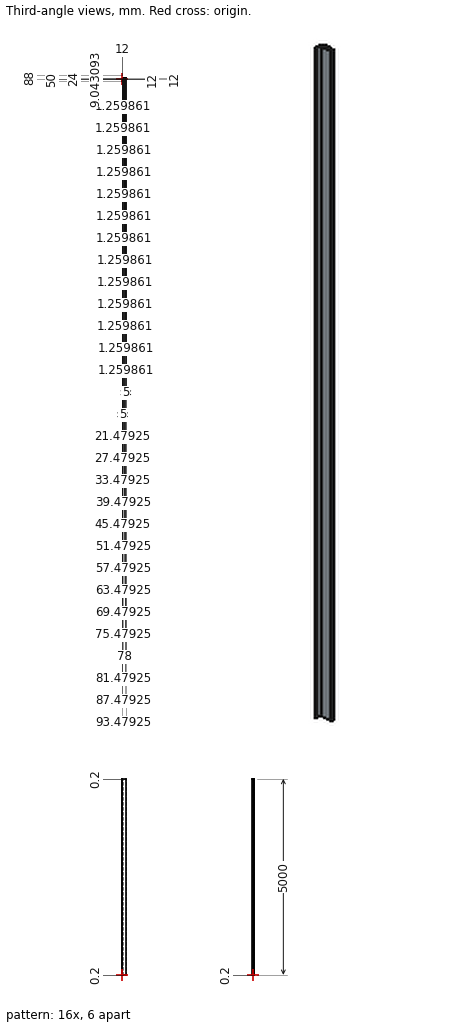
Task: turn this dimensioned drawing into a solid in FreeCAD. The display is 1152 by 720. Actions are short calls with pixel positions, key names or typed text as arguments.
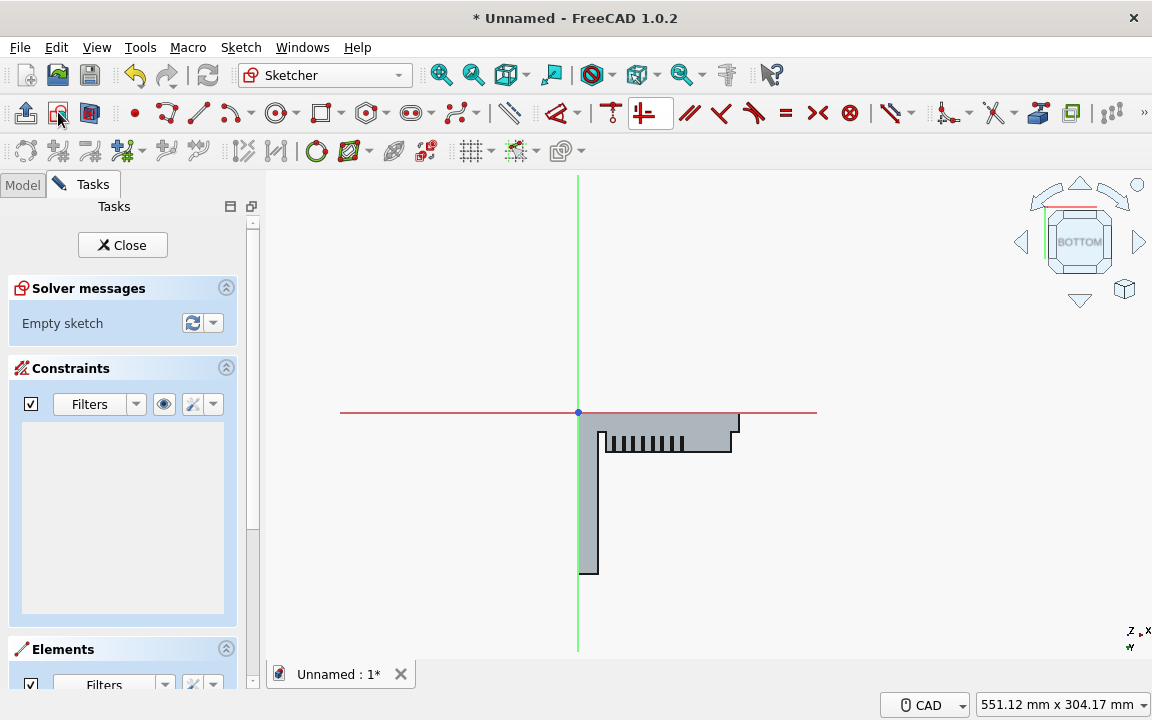
scroll(694, 446, up, 15)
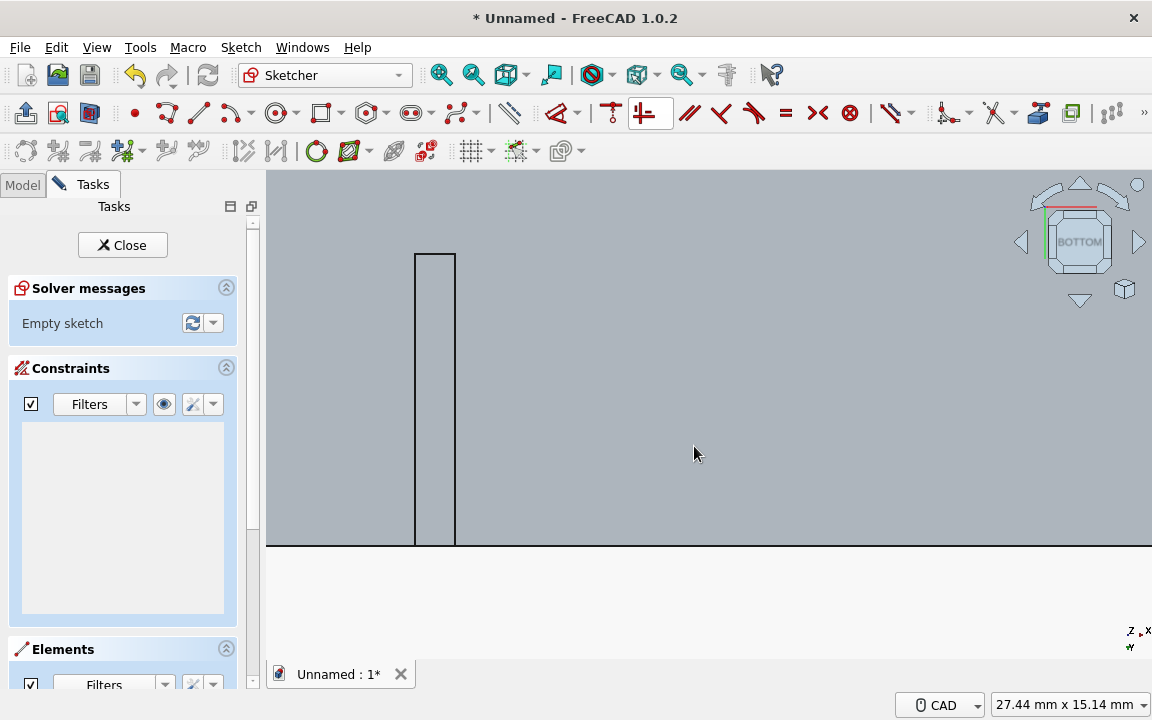
click(322, 114)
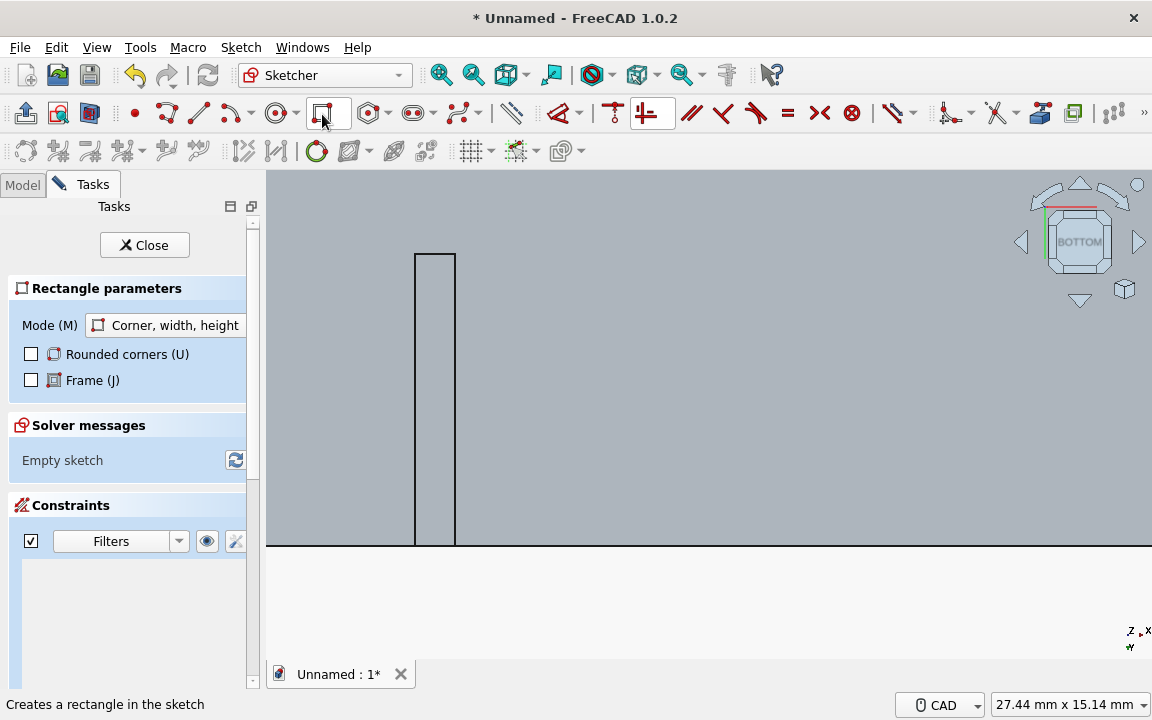
click(608, 254)
click(649, 546)
key(Escape)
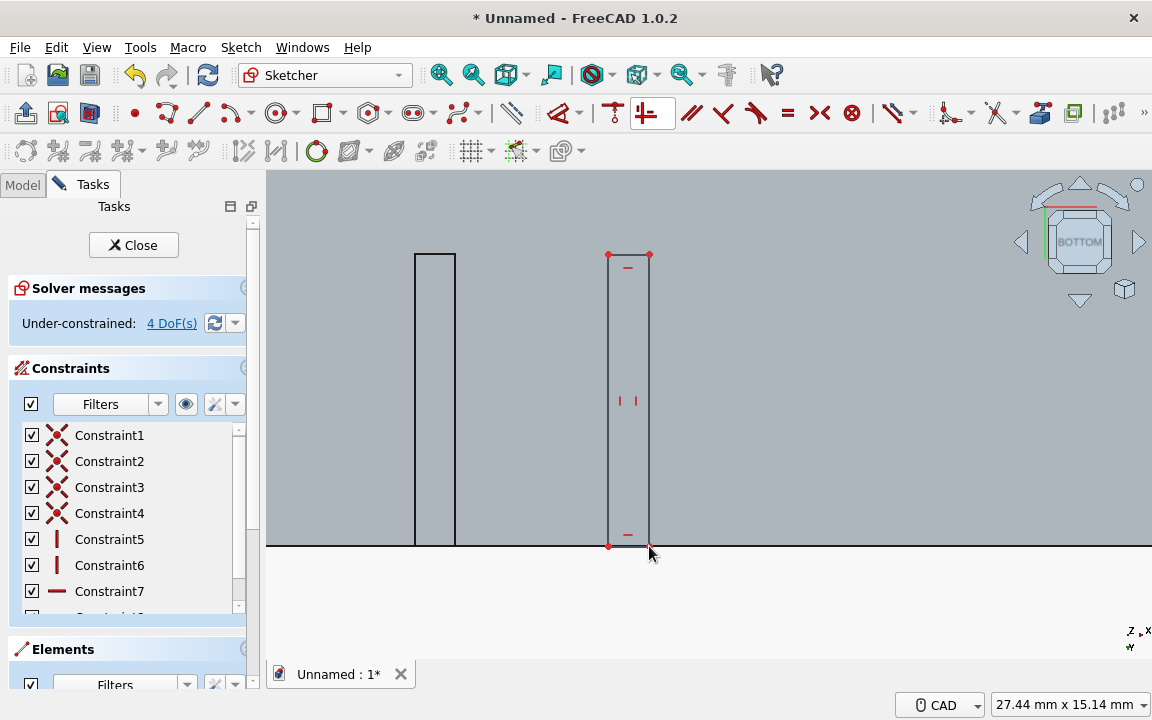
click(558, 114)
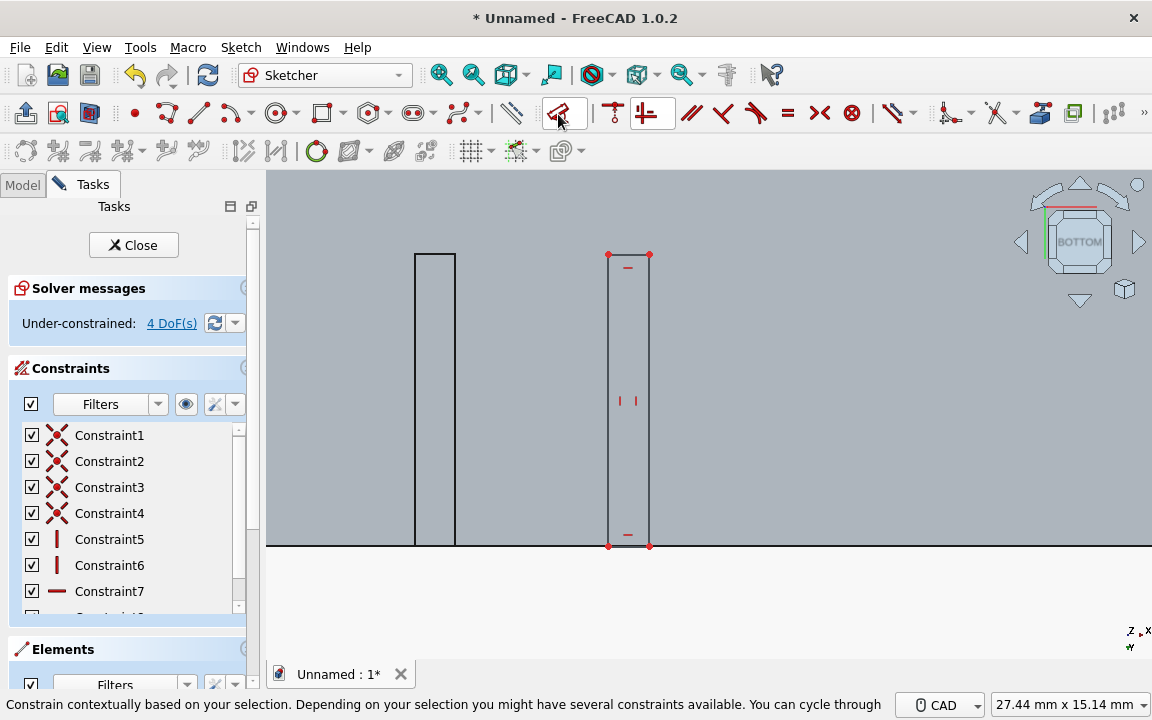
click(608, 547)
click(666, 373)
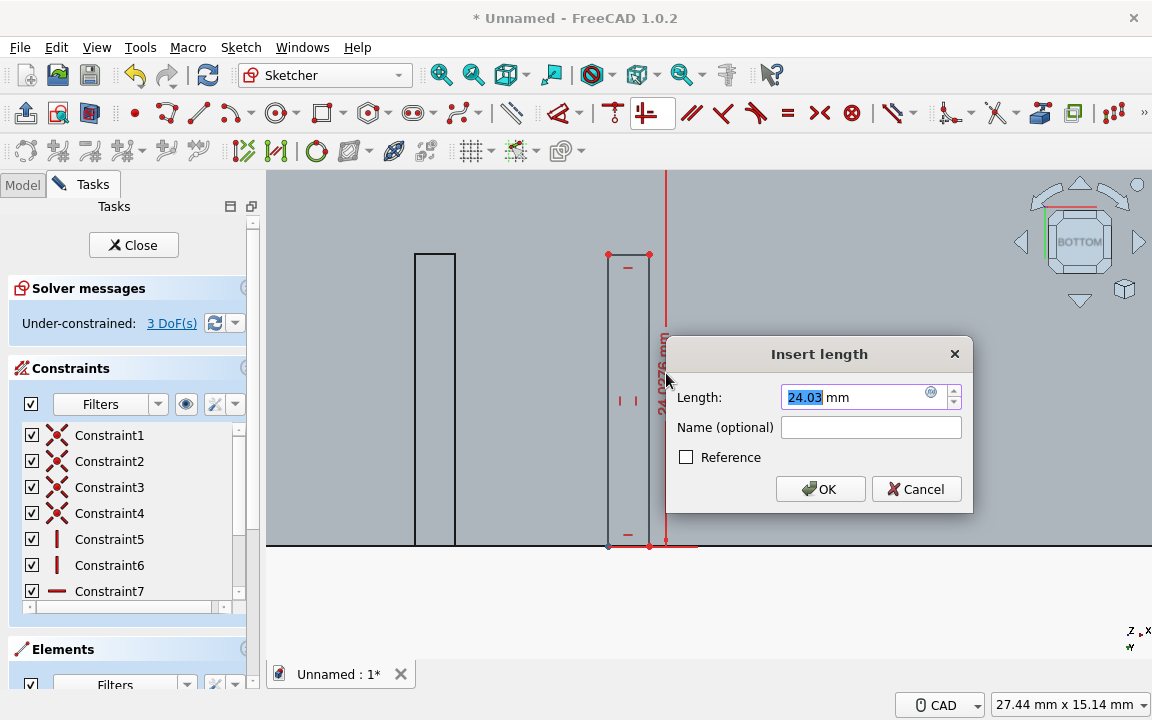
text(24)
key(Return)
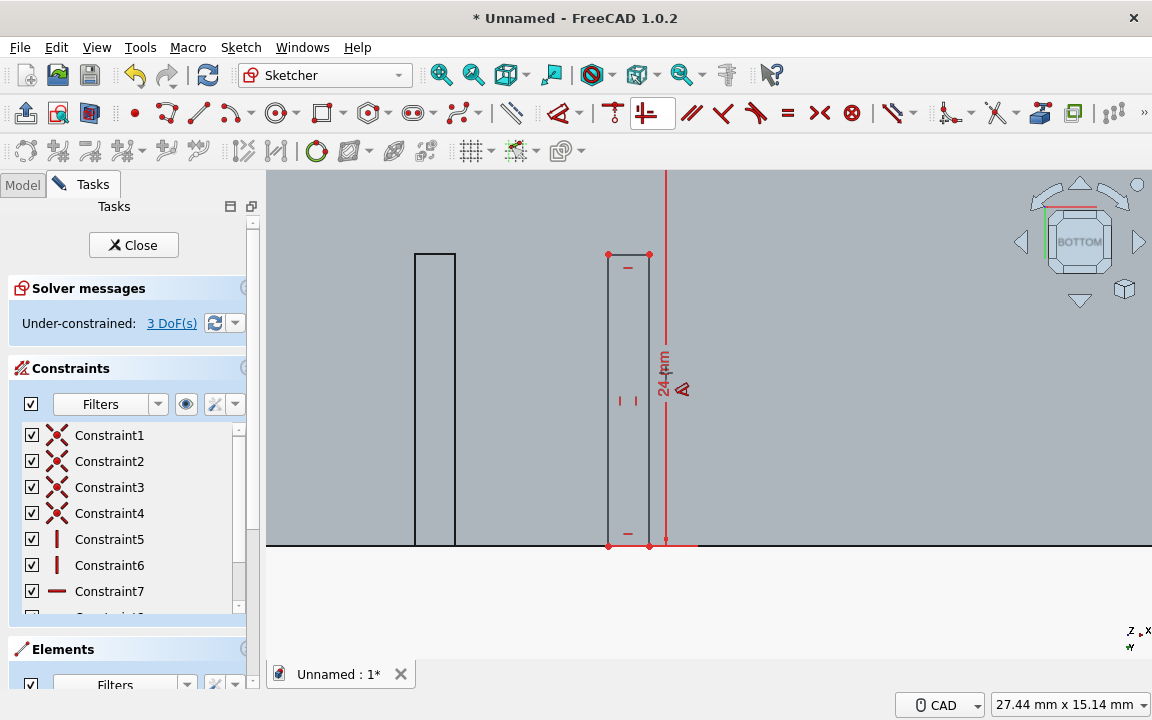
click(608, 342)
click(574, 401)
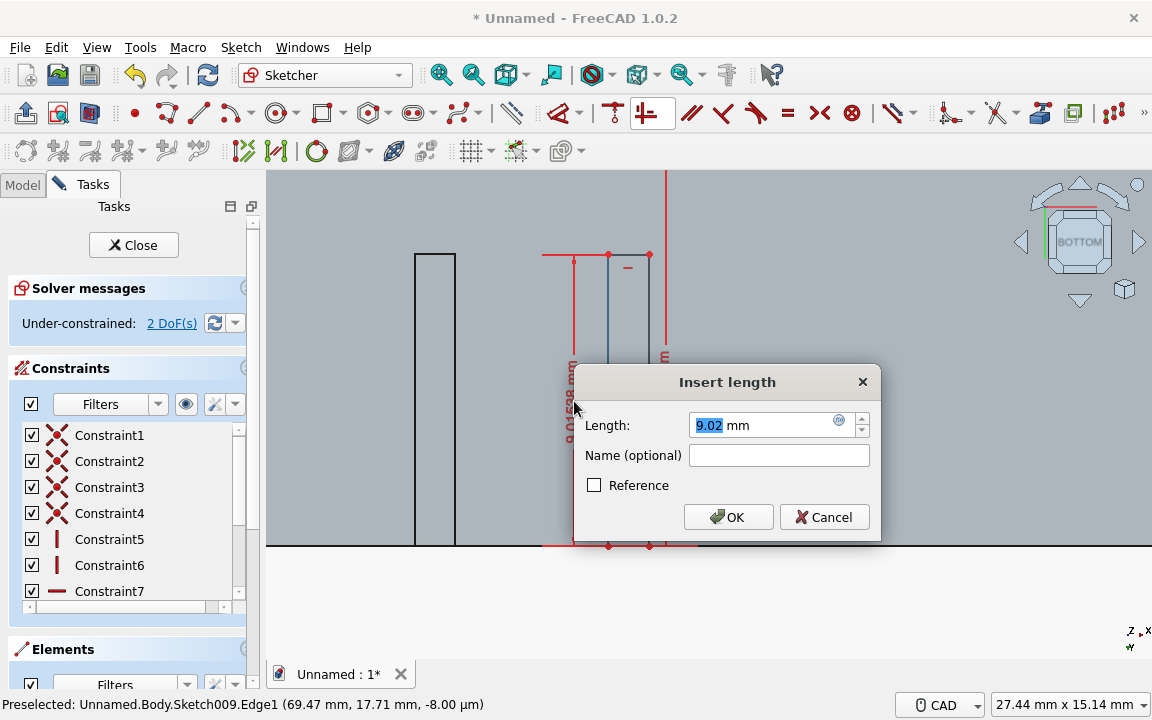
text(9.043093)
key(Return)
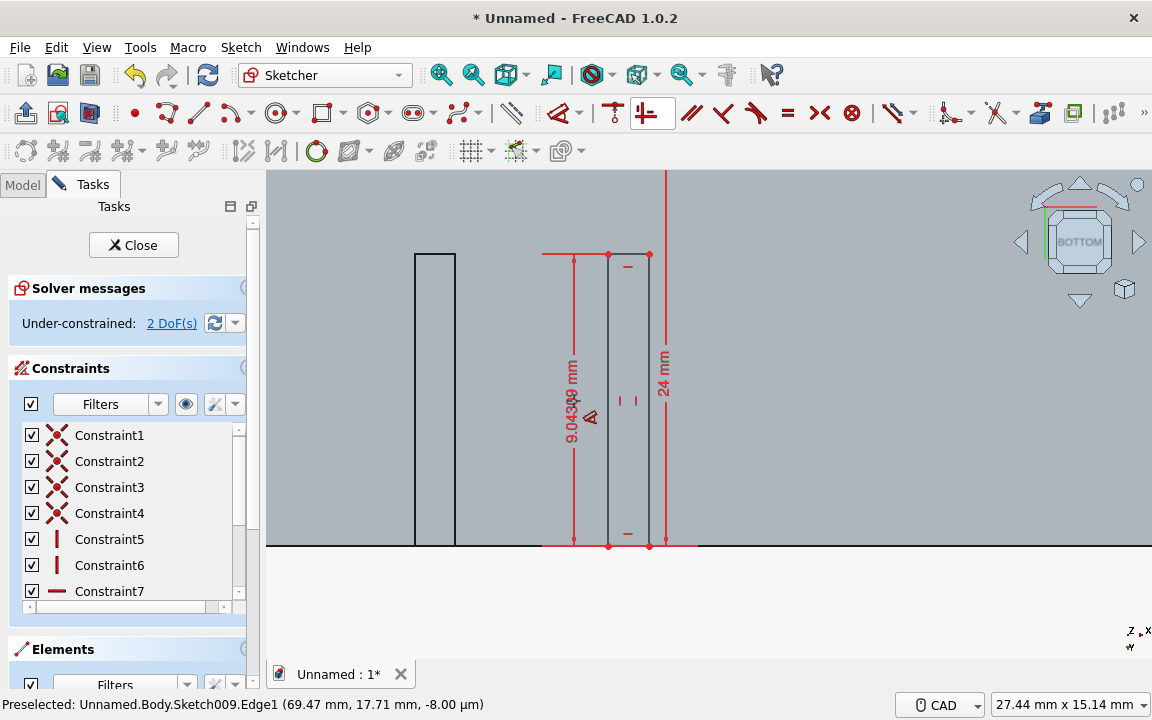
click(620, 546)
click(628, 580)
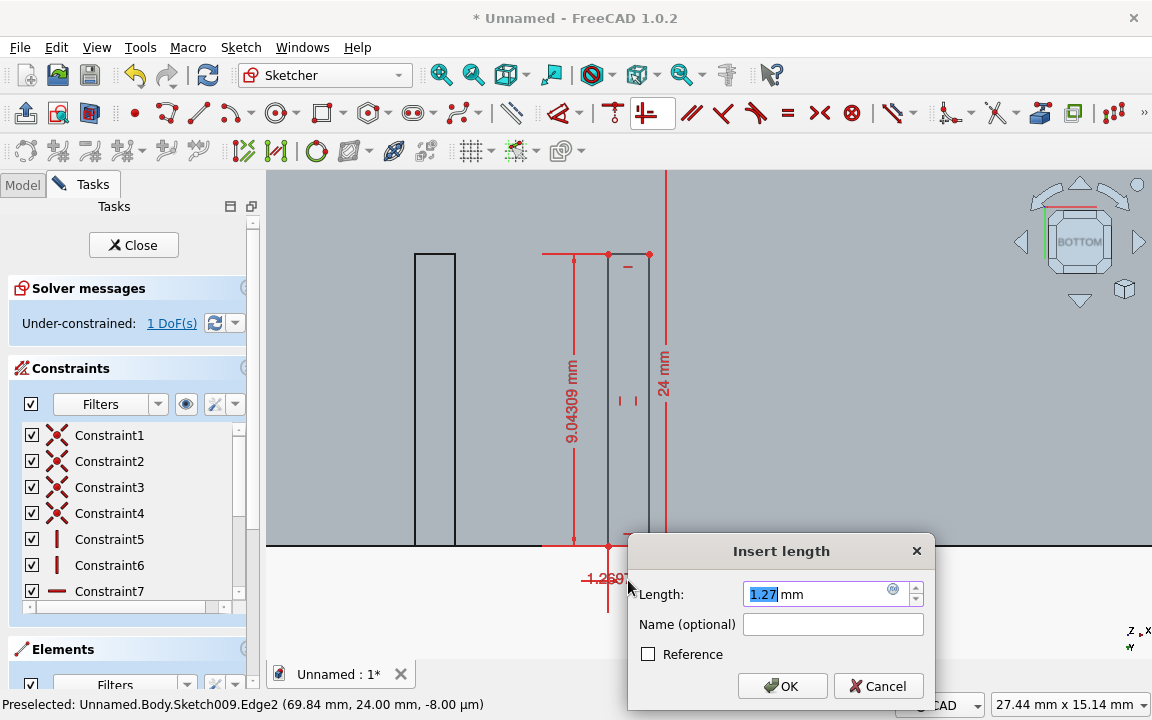
text(1.259861)
key(Return)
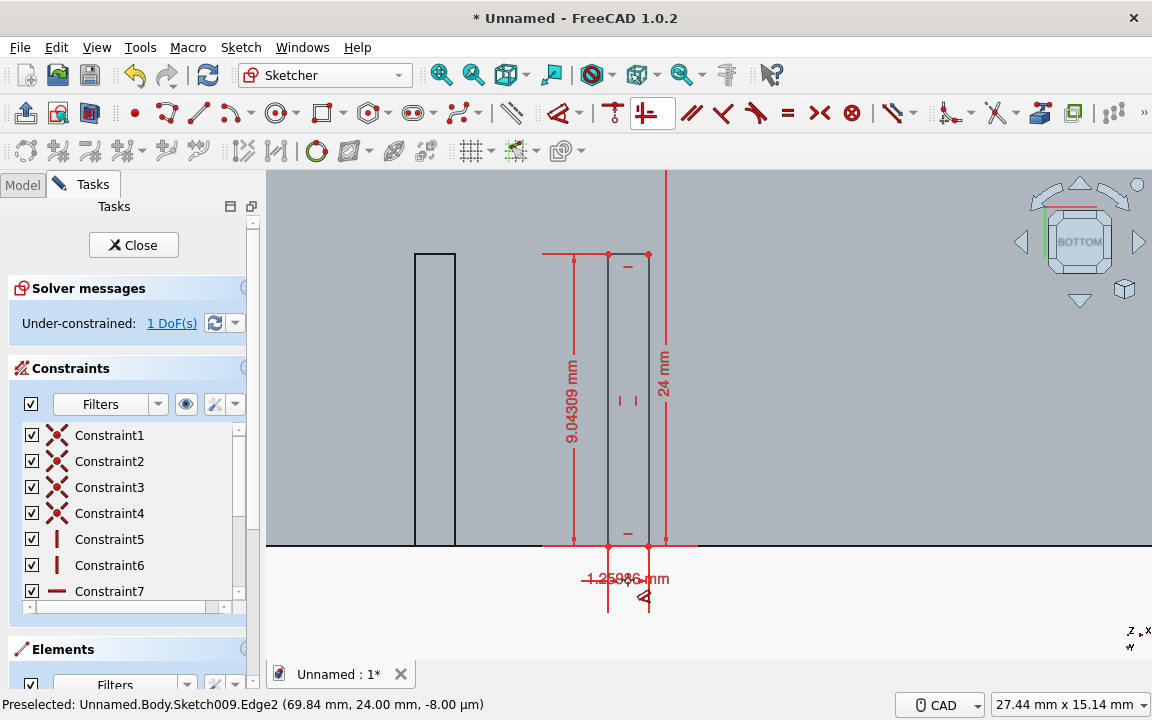
click(608, 254)
click(451, 288)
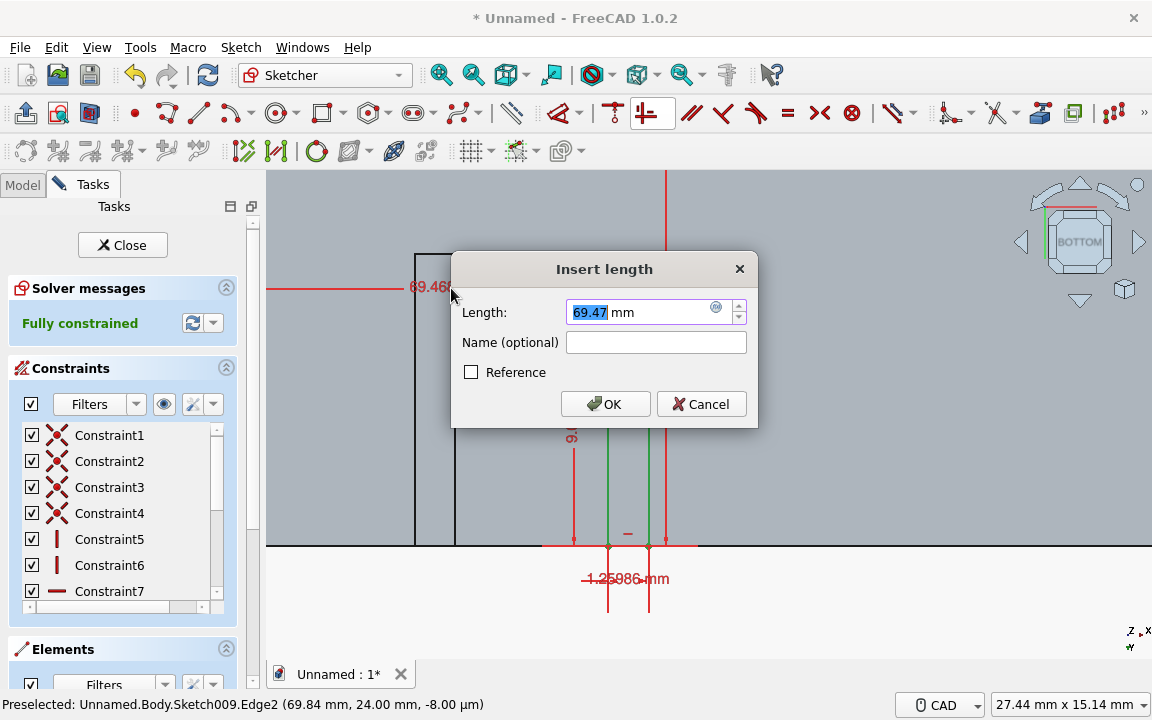
text(69.47925)
key(Return)
key(Escape)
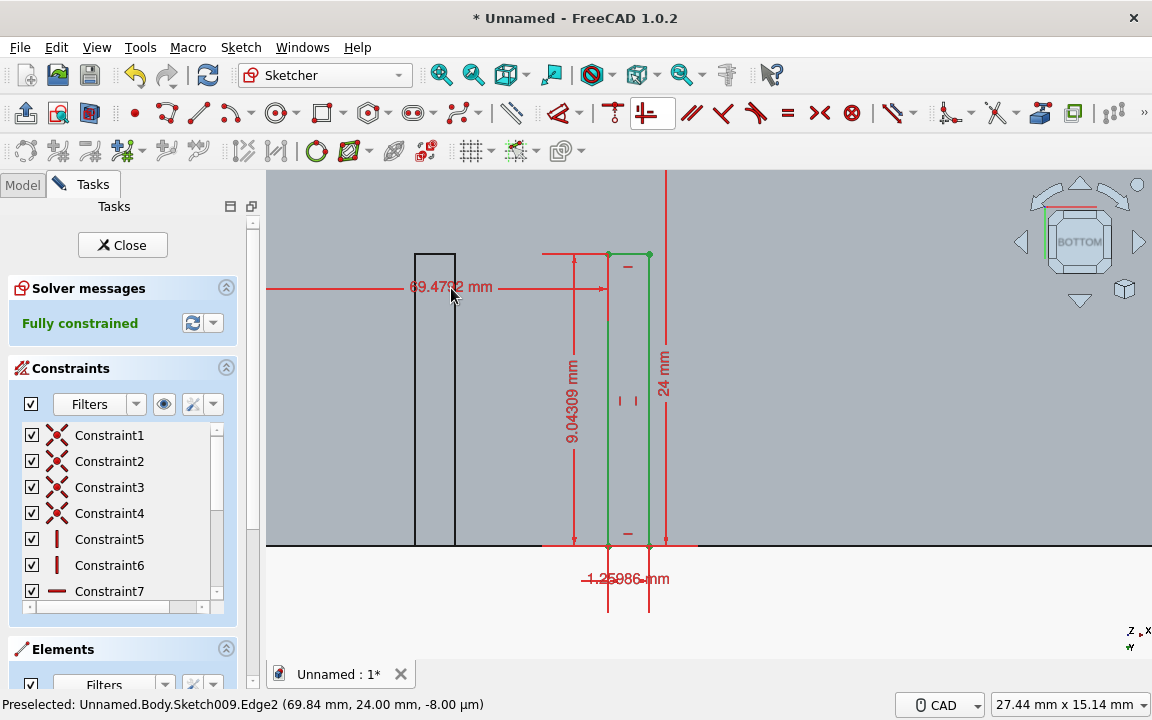
click(123, 245)